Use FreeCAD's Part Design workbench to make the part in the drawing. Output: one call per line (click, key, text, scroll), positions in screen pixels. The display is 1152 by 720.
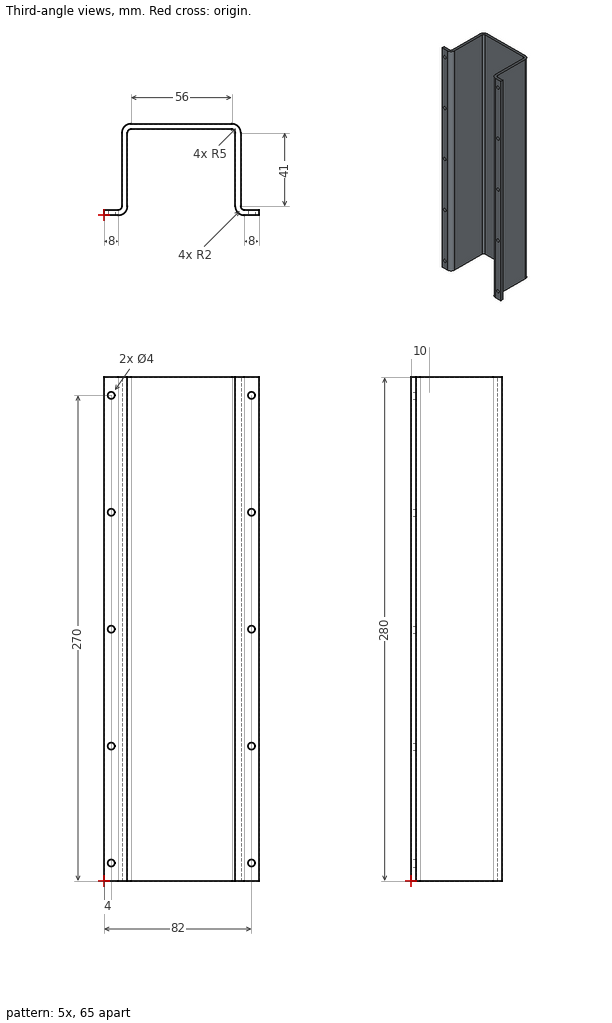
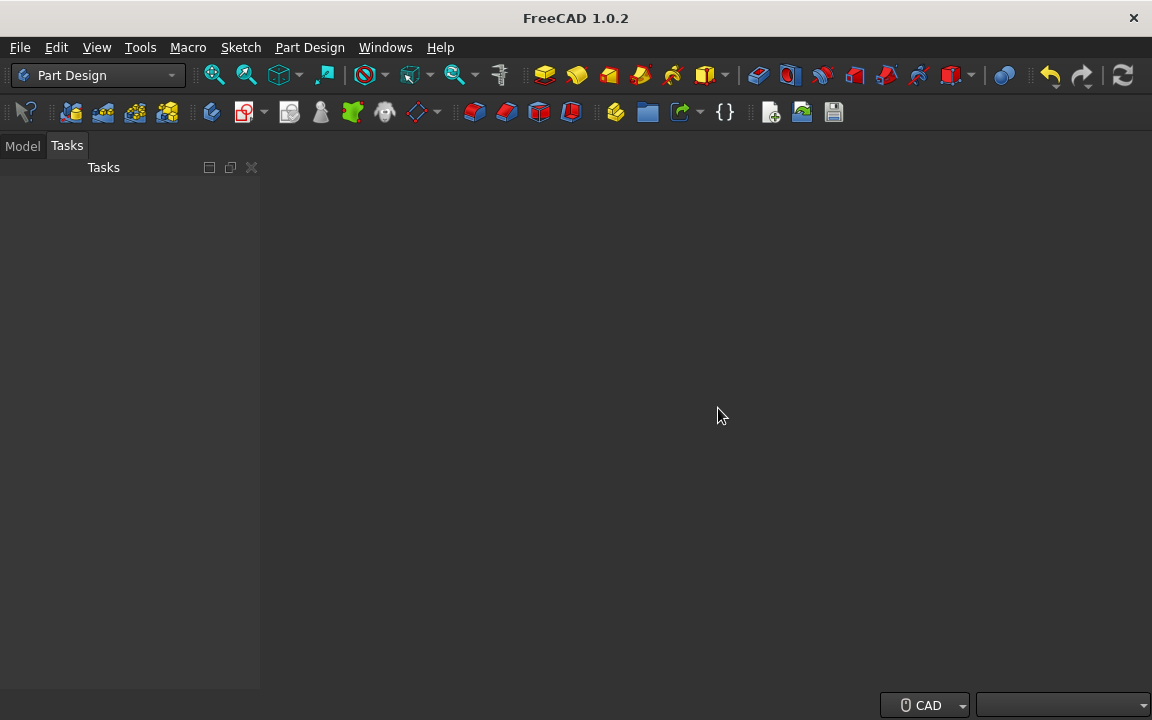
key(ctrl+n)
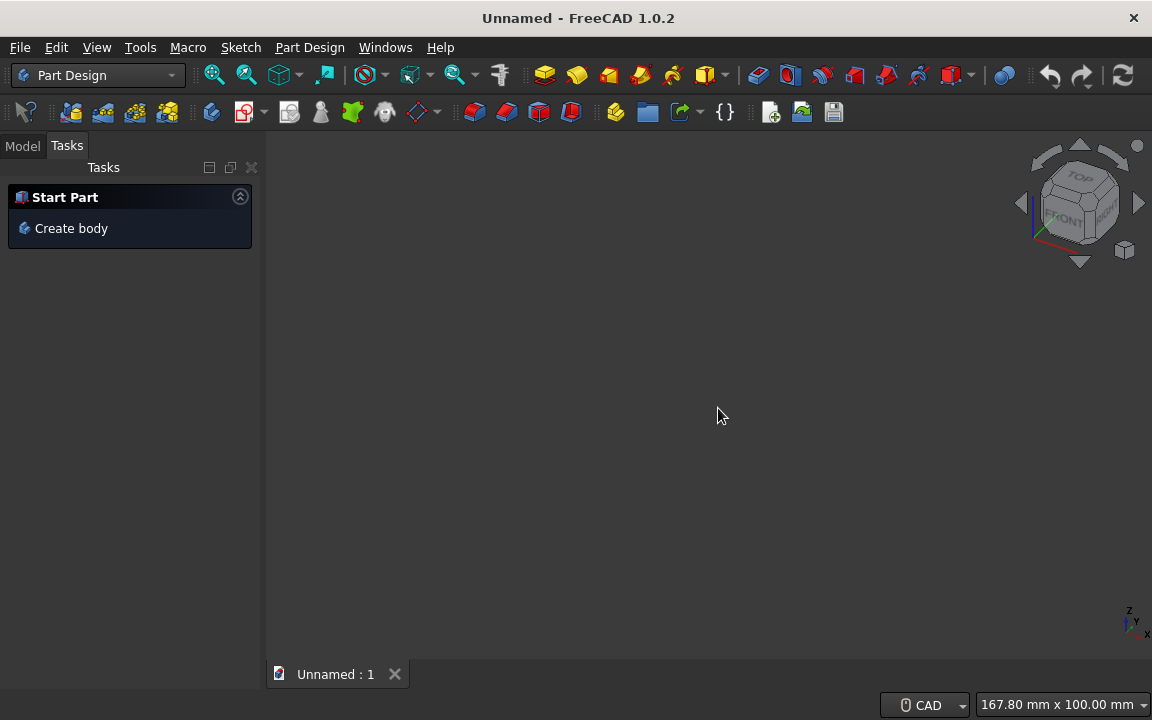
click(244, 112)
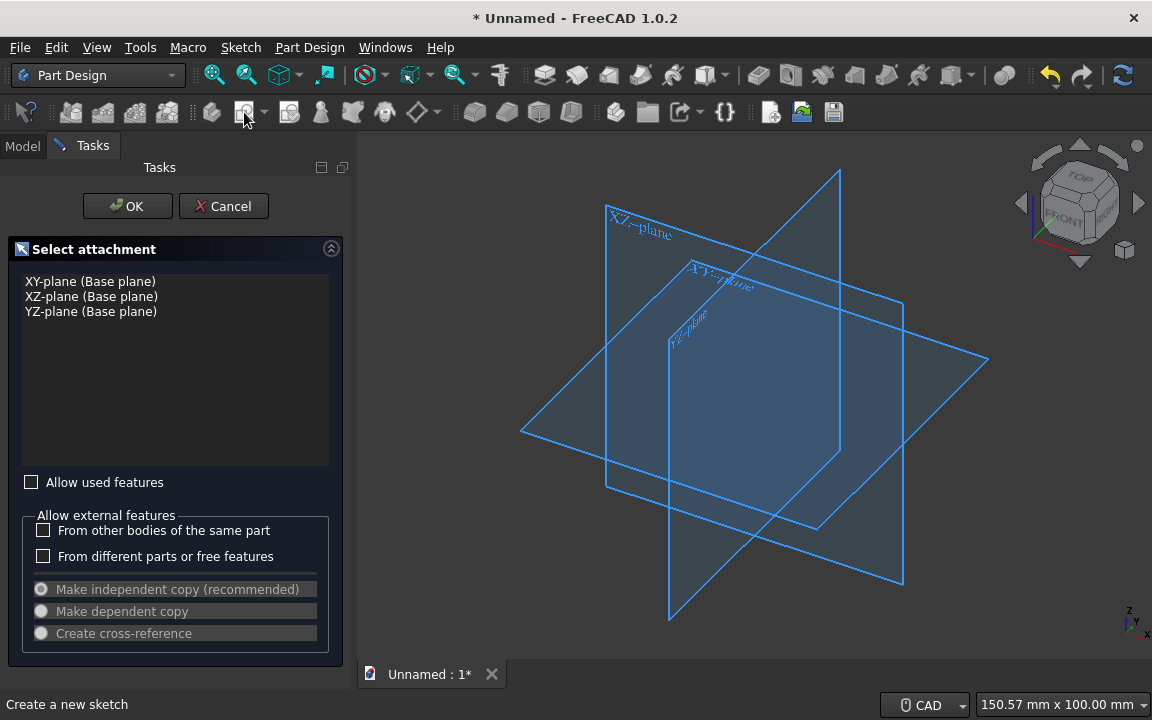
click(82, 282)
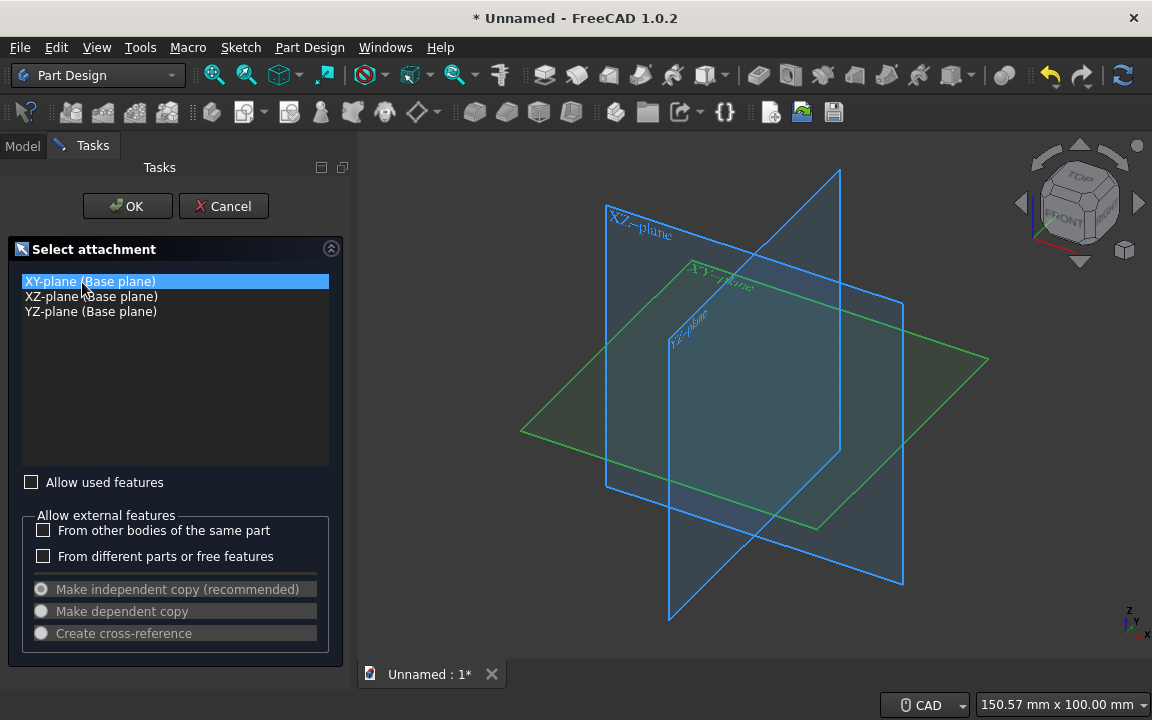
click(128, 206)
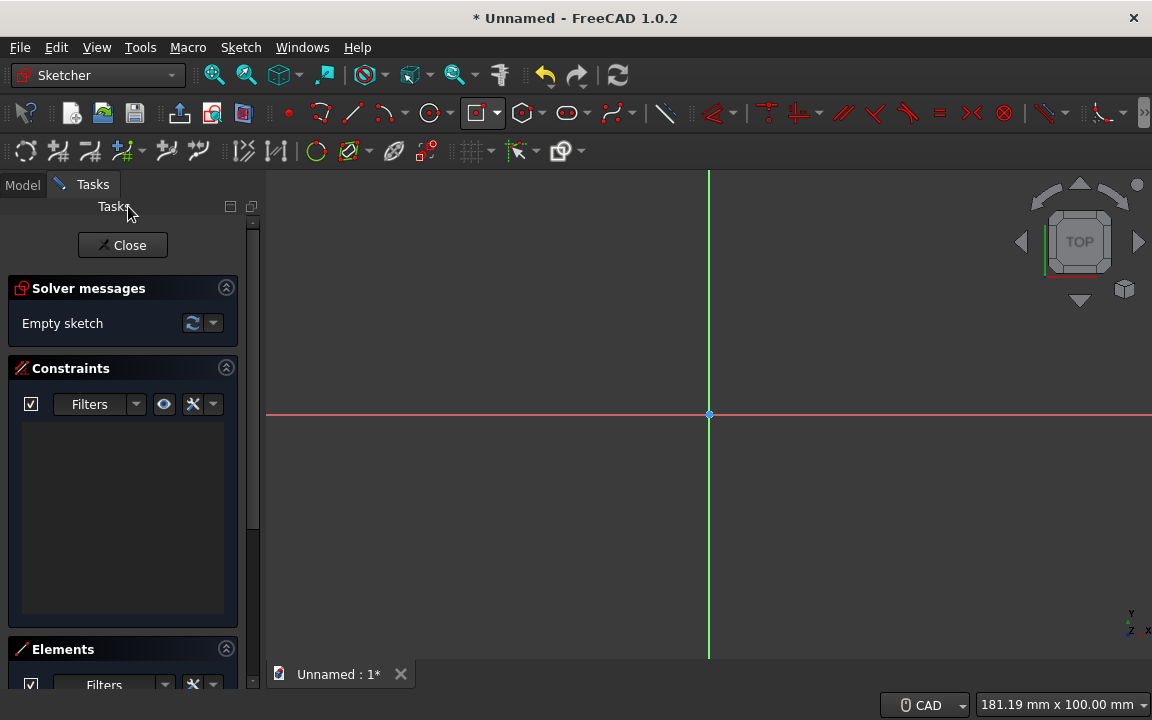
scroll(294, 631, down, 2)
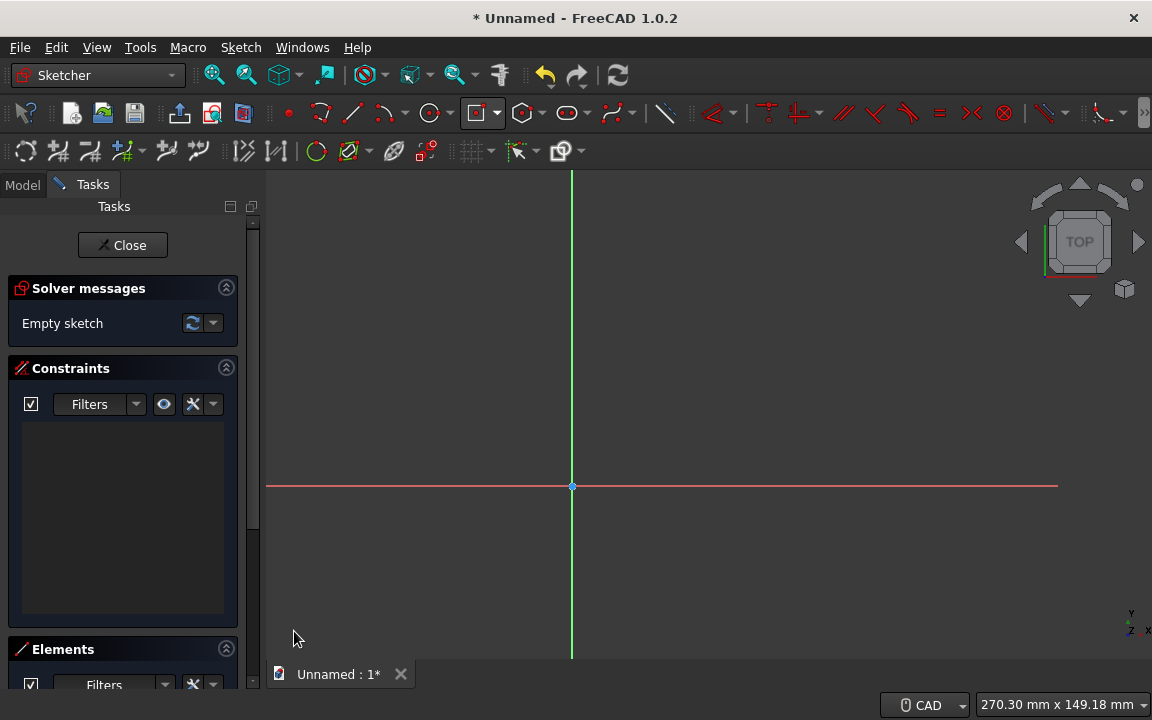
scroll(802, 388, up, 3)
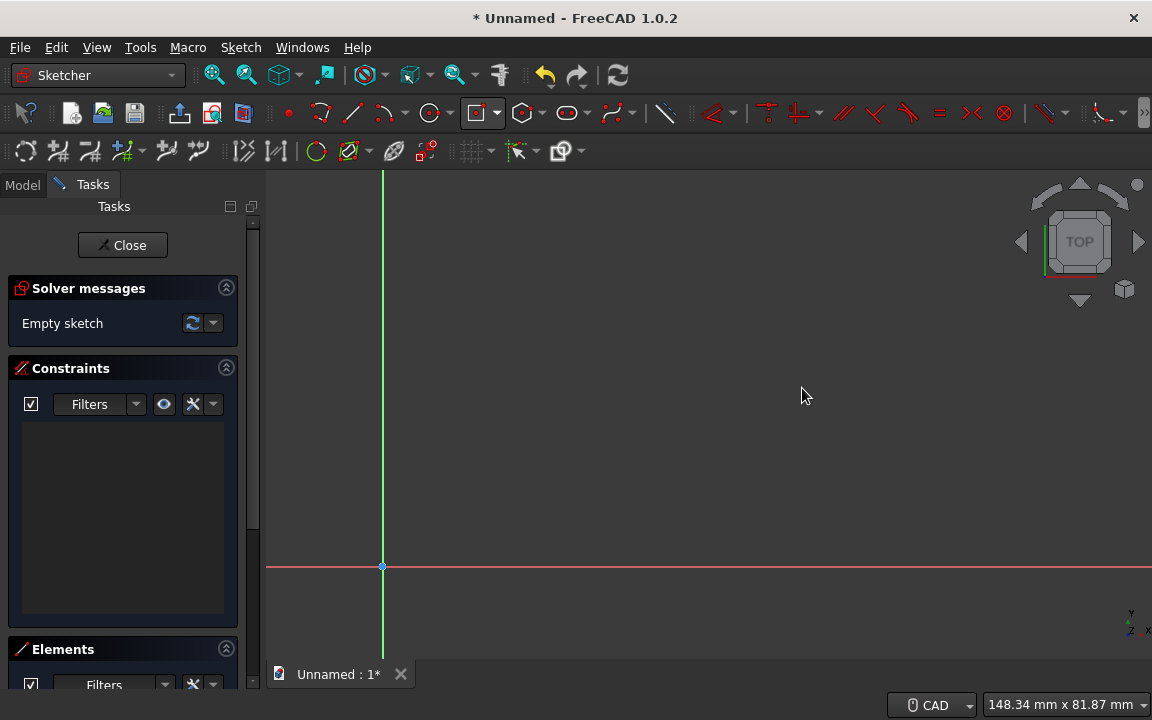
click(354, 114)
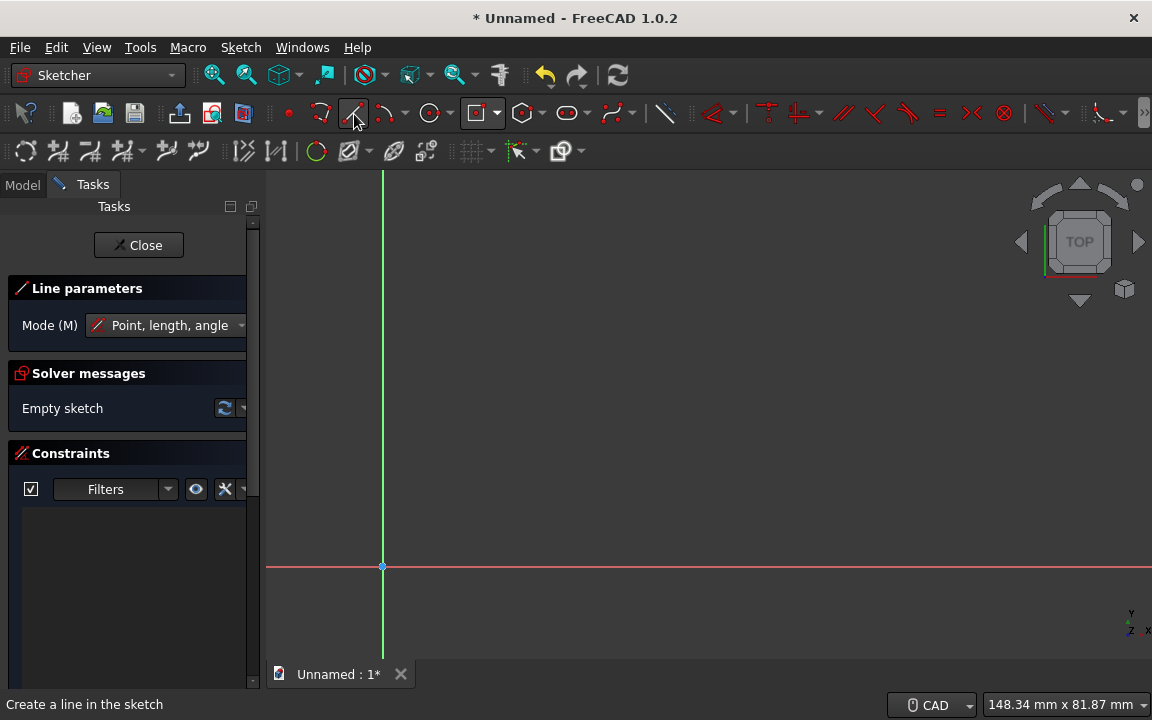
click(837, 537)
click(837, 292)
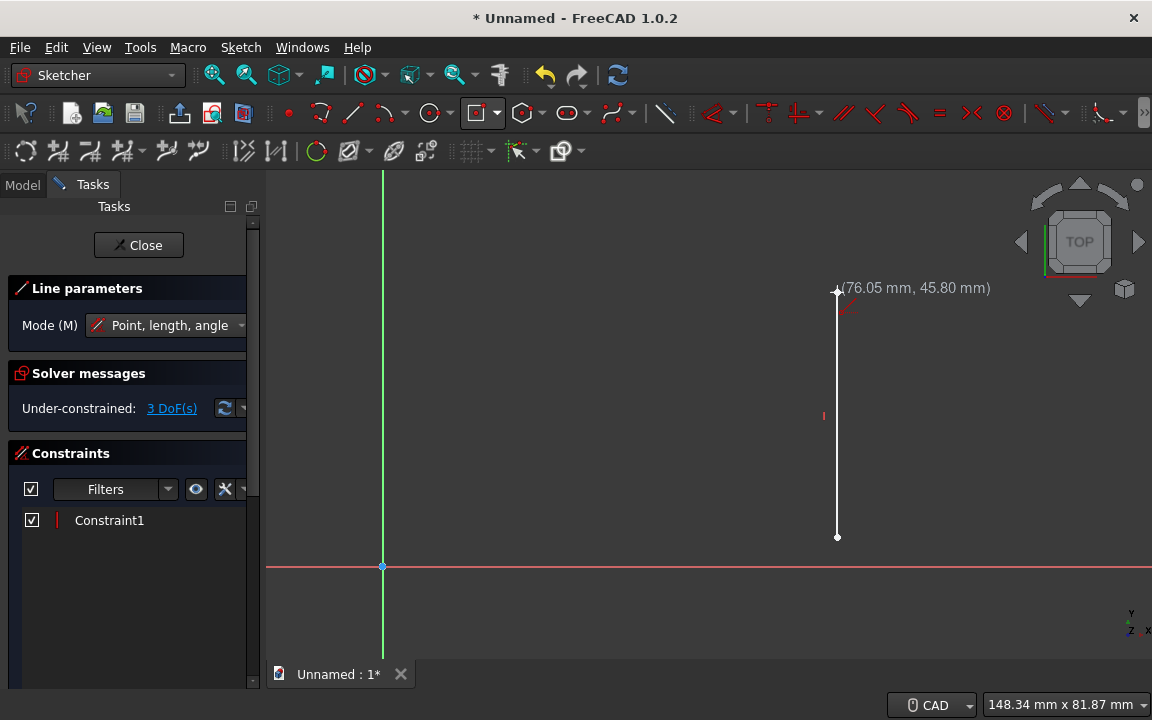
click(807, 262)
click(472, 262)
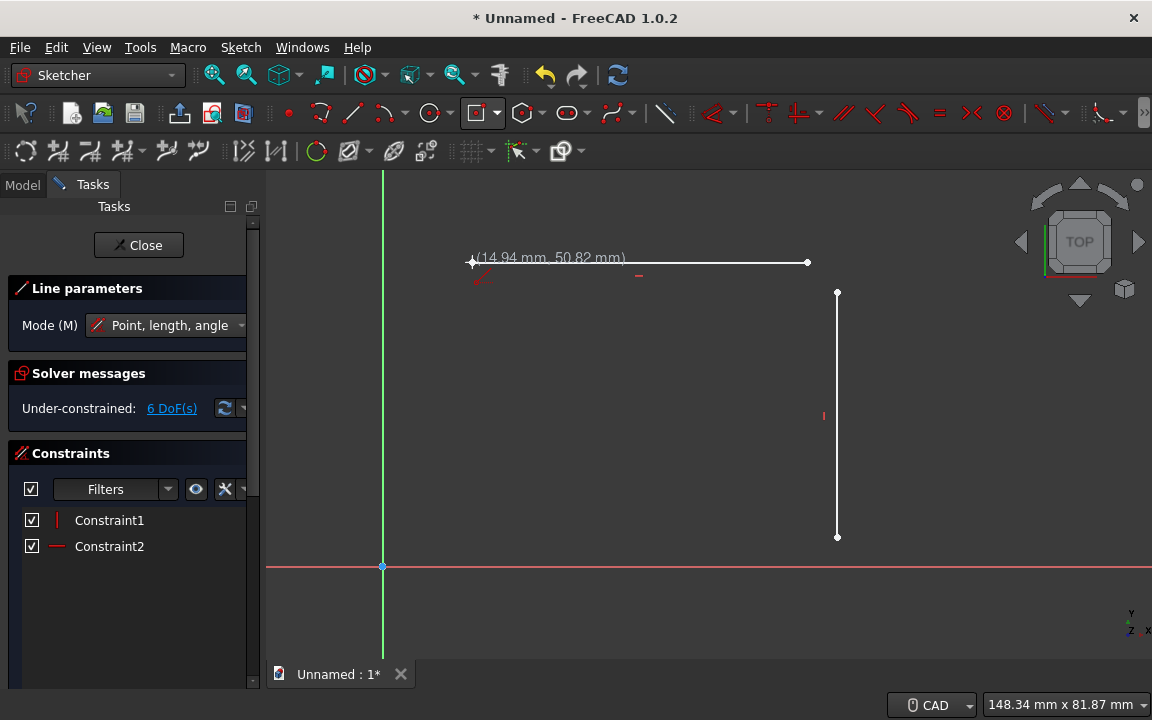
click(442, 292)
click(442, 537)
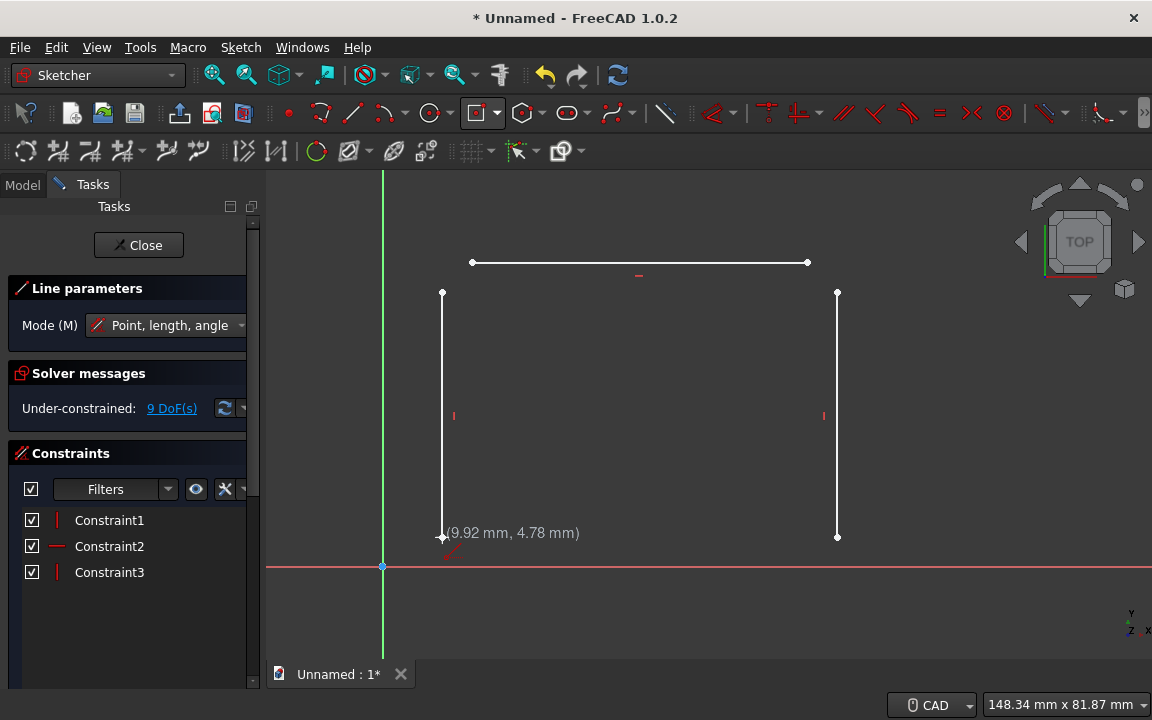
click(322, 114)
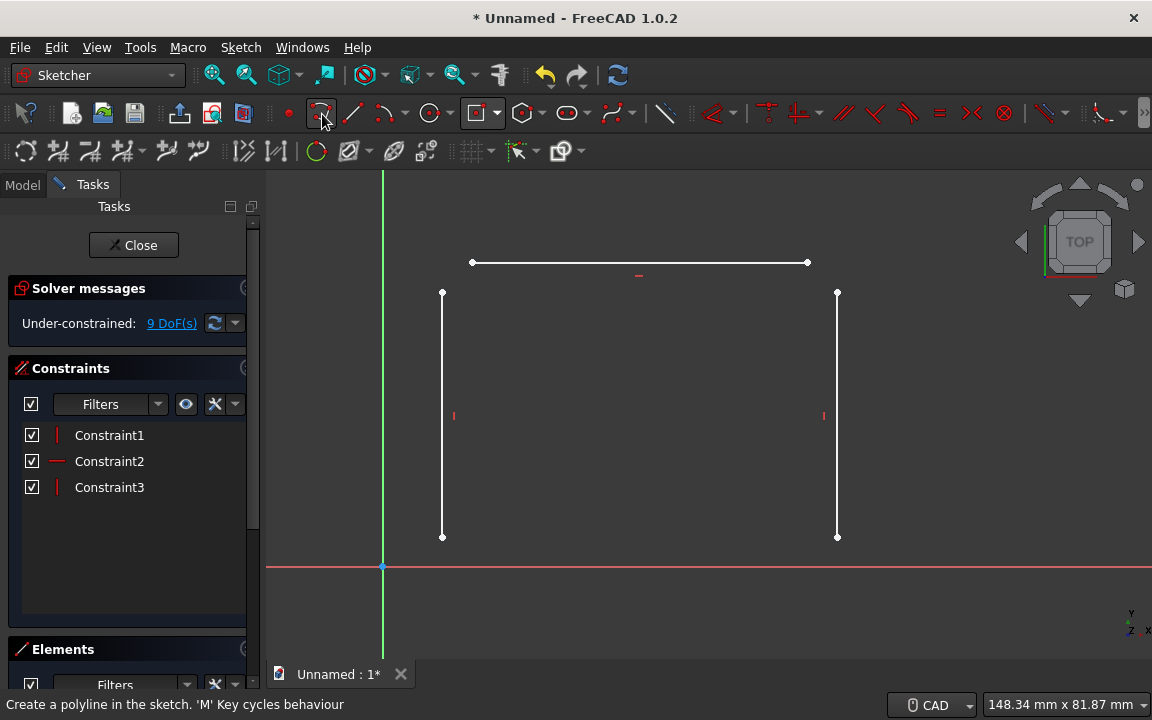
click(431, 549)
click(383, 549)
click(383, 567)
click(431, 558)
right_click(431, 558)